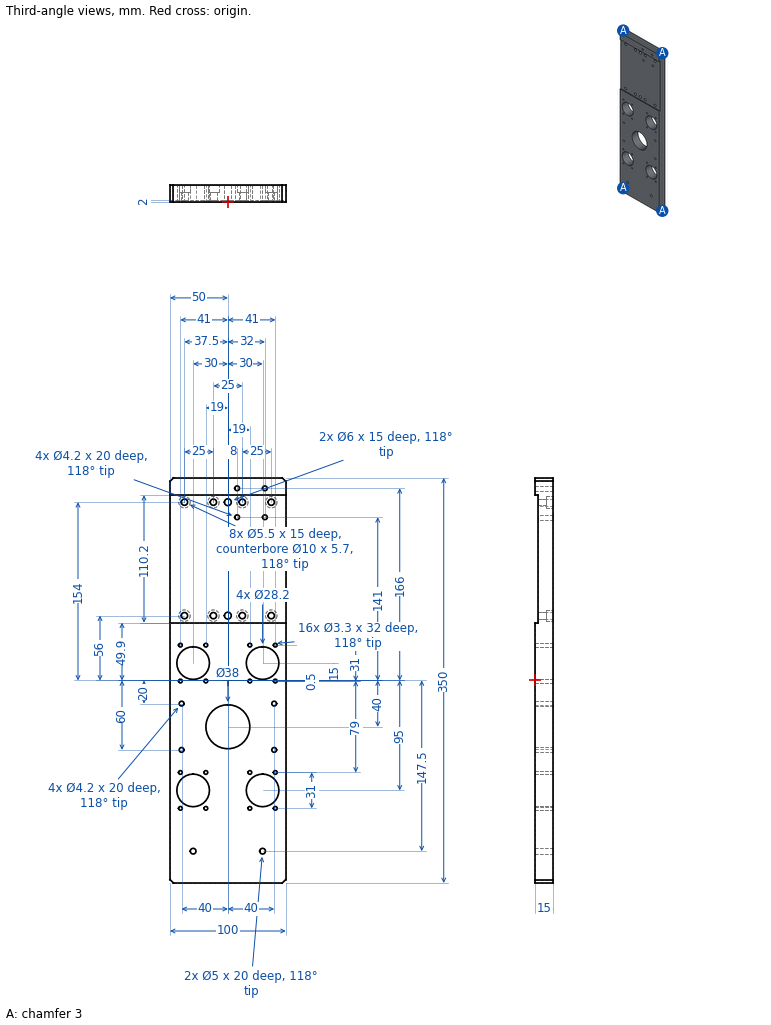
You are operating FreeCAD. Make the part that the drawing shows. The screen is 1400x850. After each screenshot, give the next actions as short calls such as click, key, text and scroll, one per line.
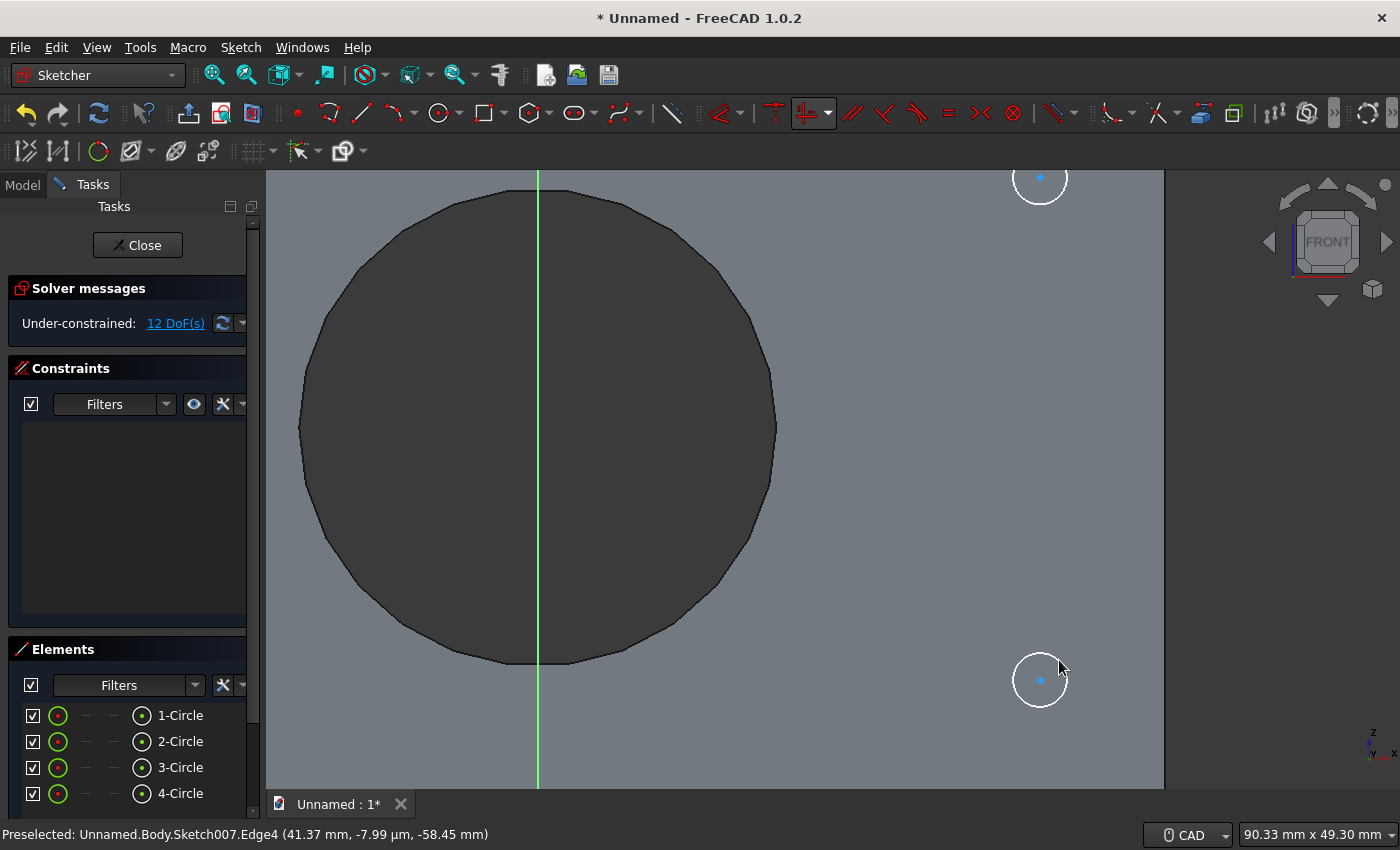
scroll(1040, 679, down, 3)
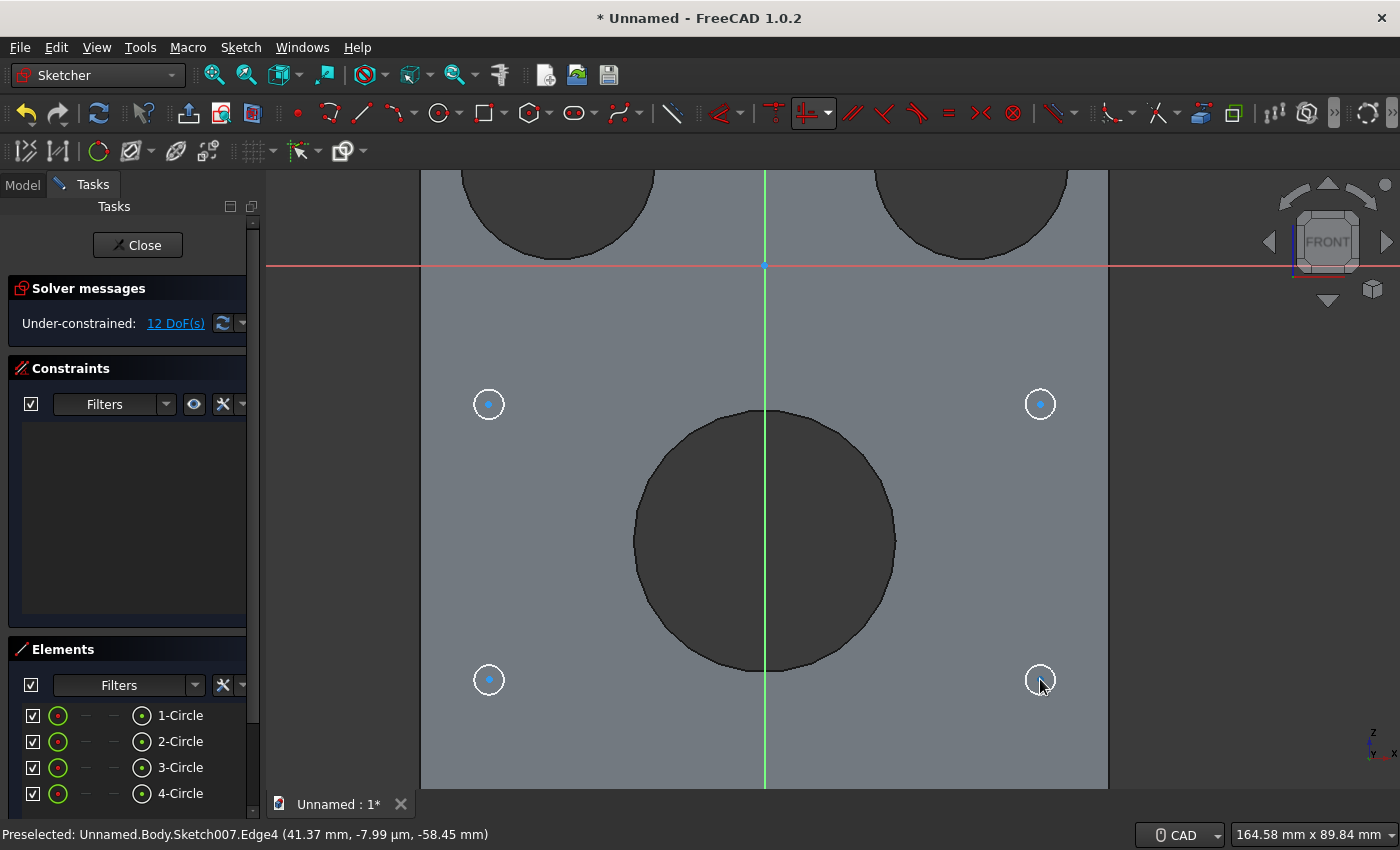
click(499, 394)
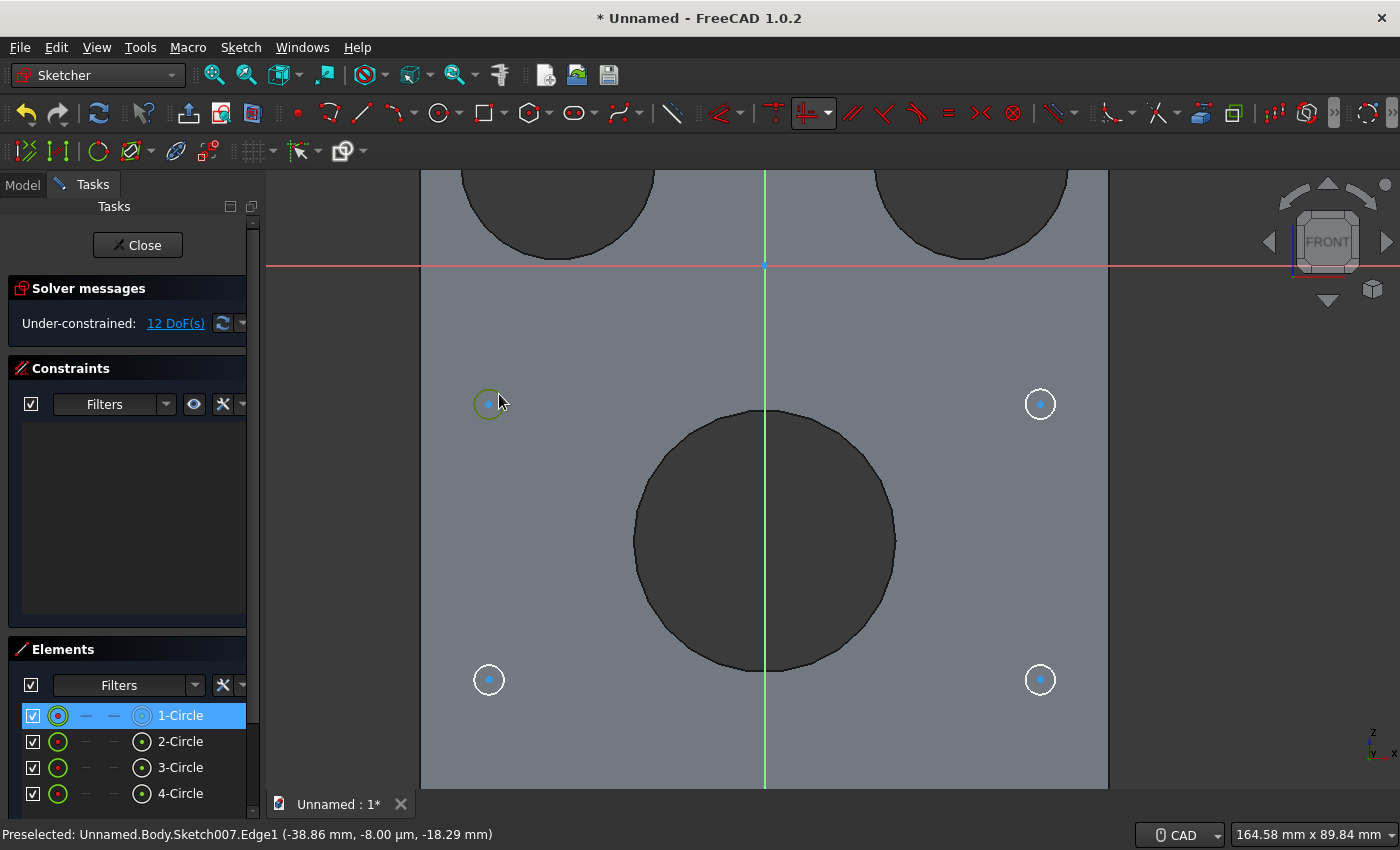
click(1051, 394)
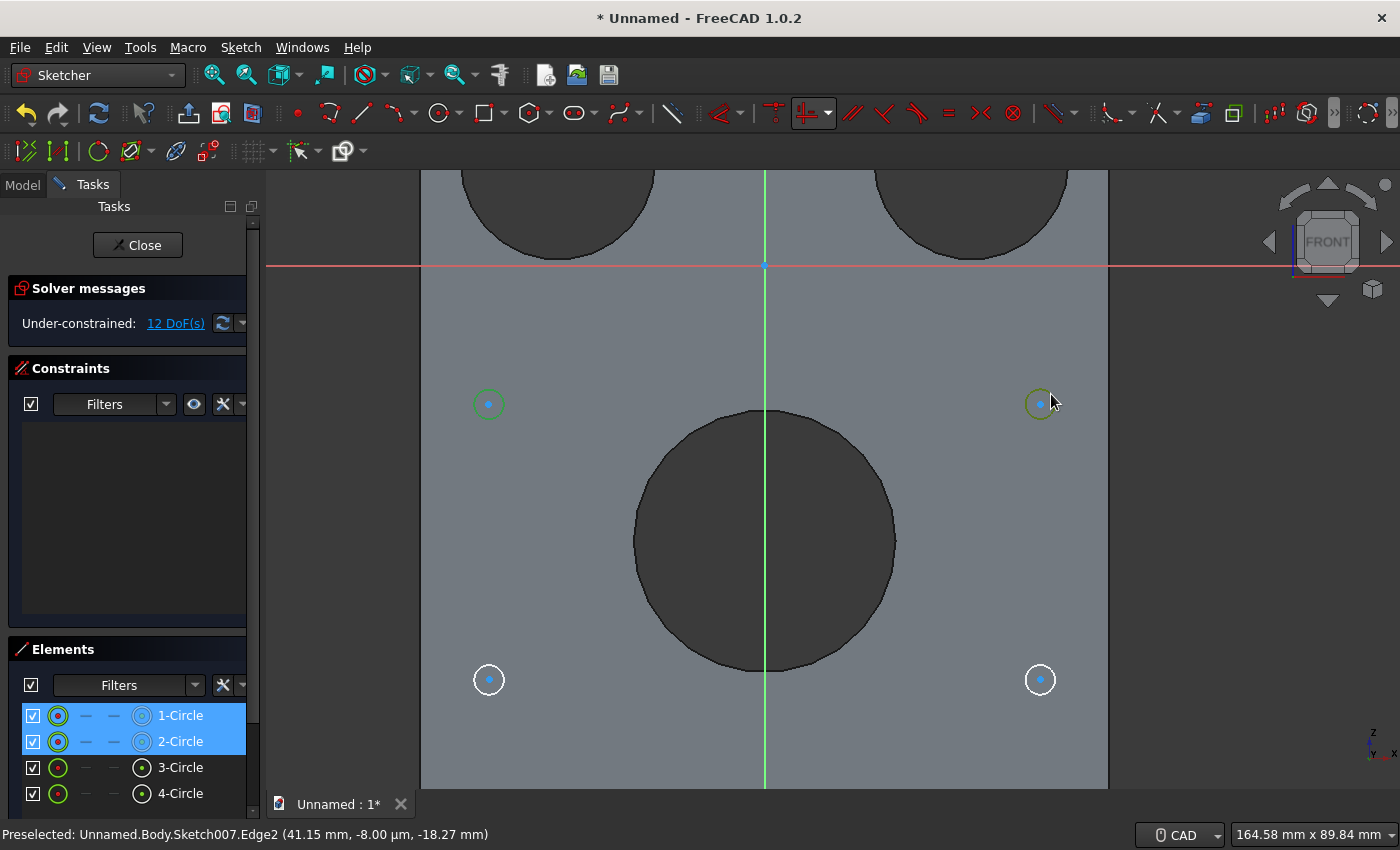
click(499, 669)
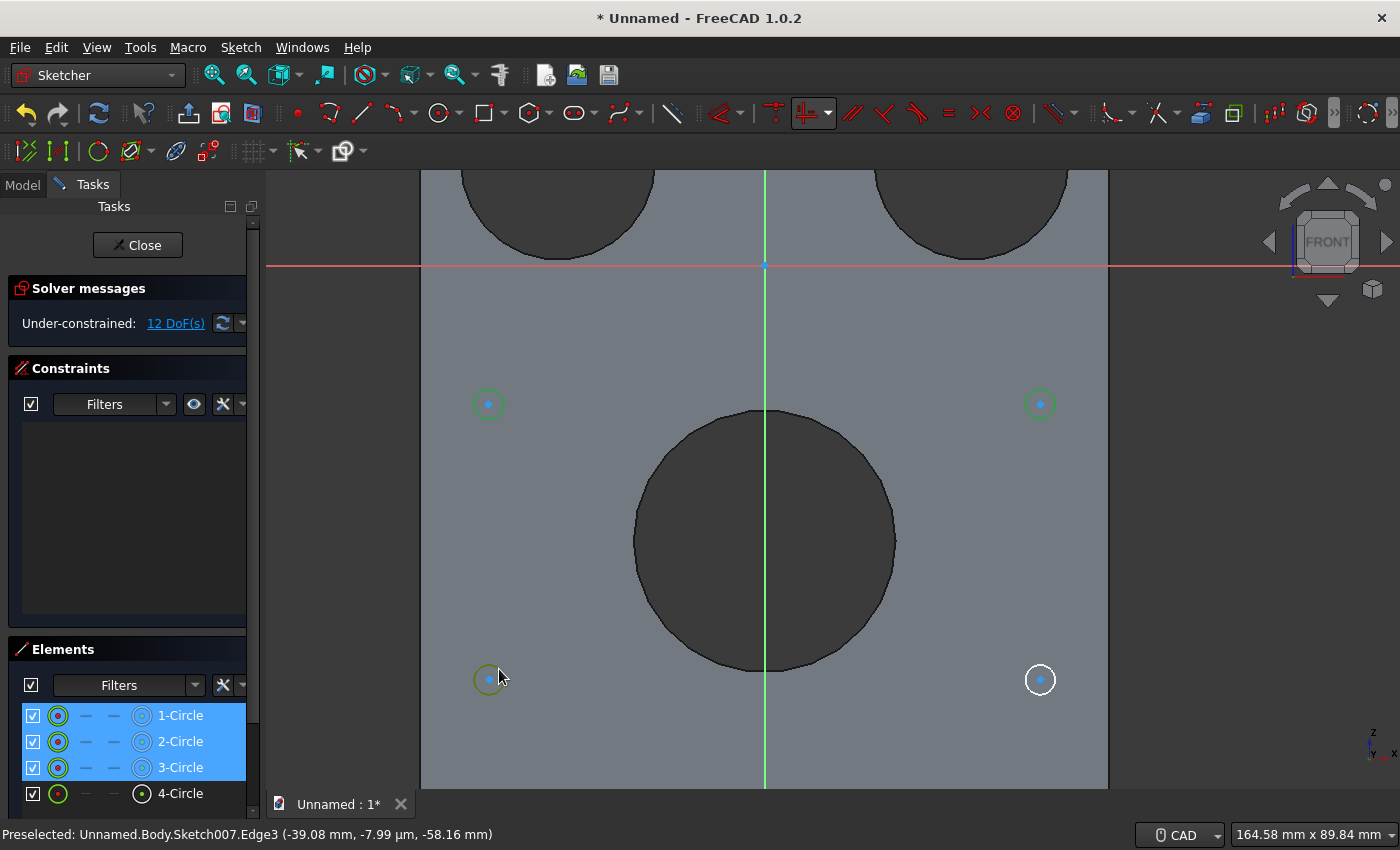
click(1051, 669)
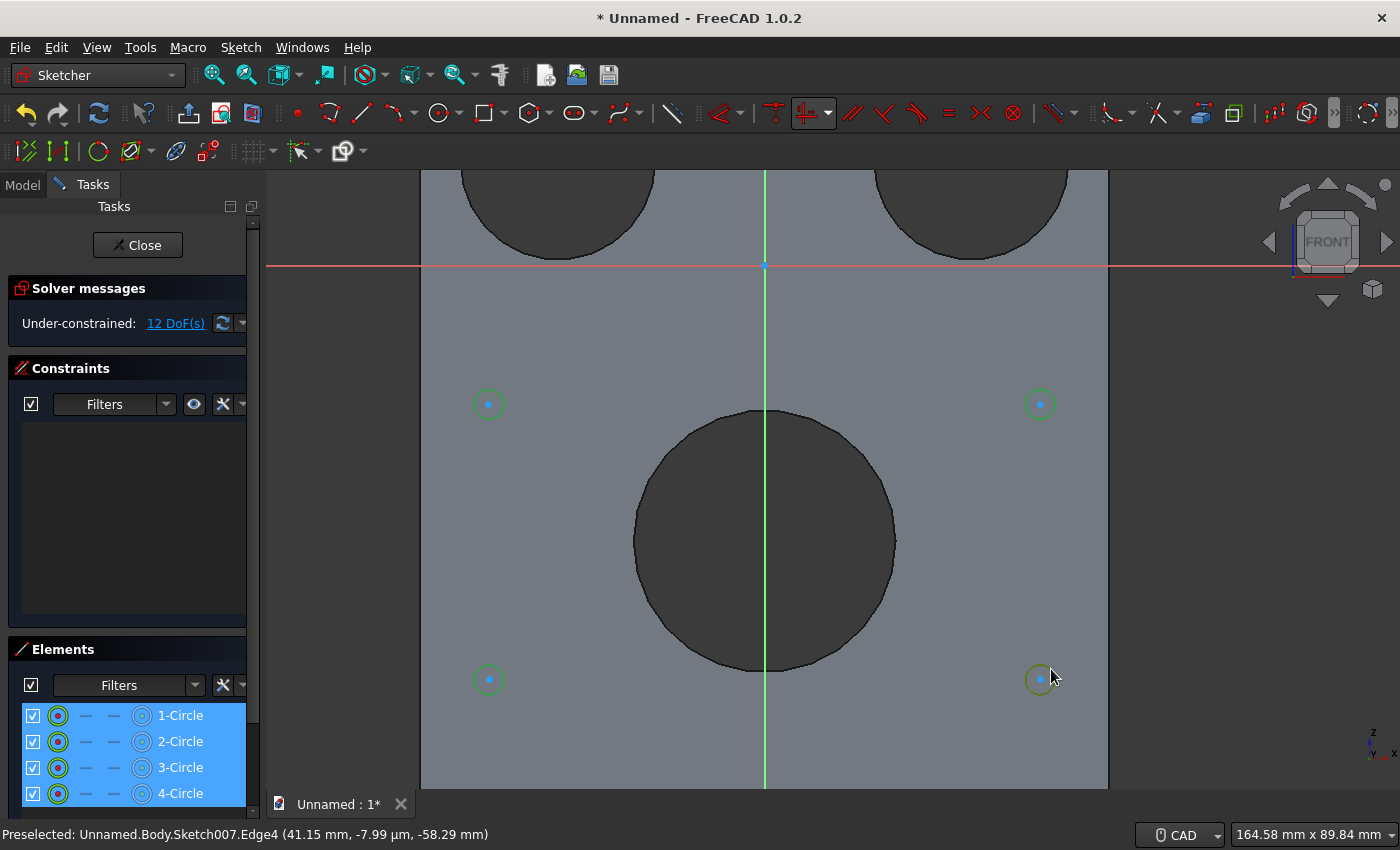
key(e)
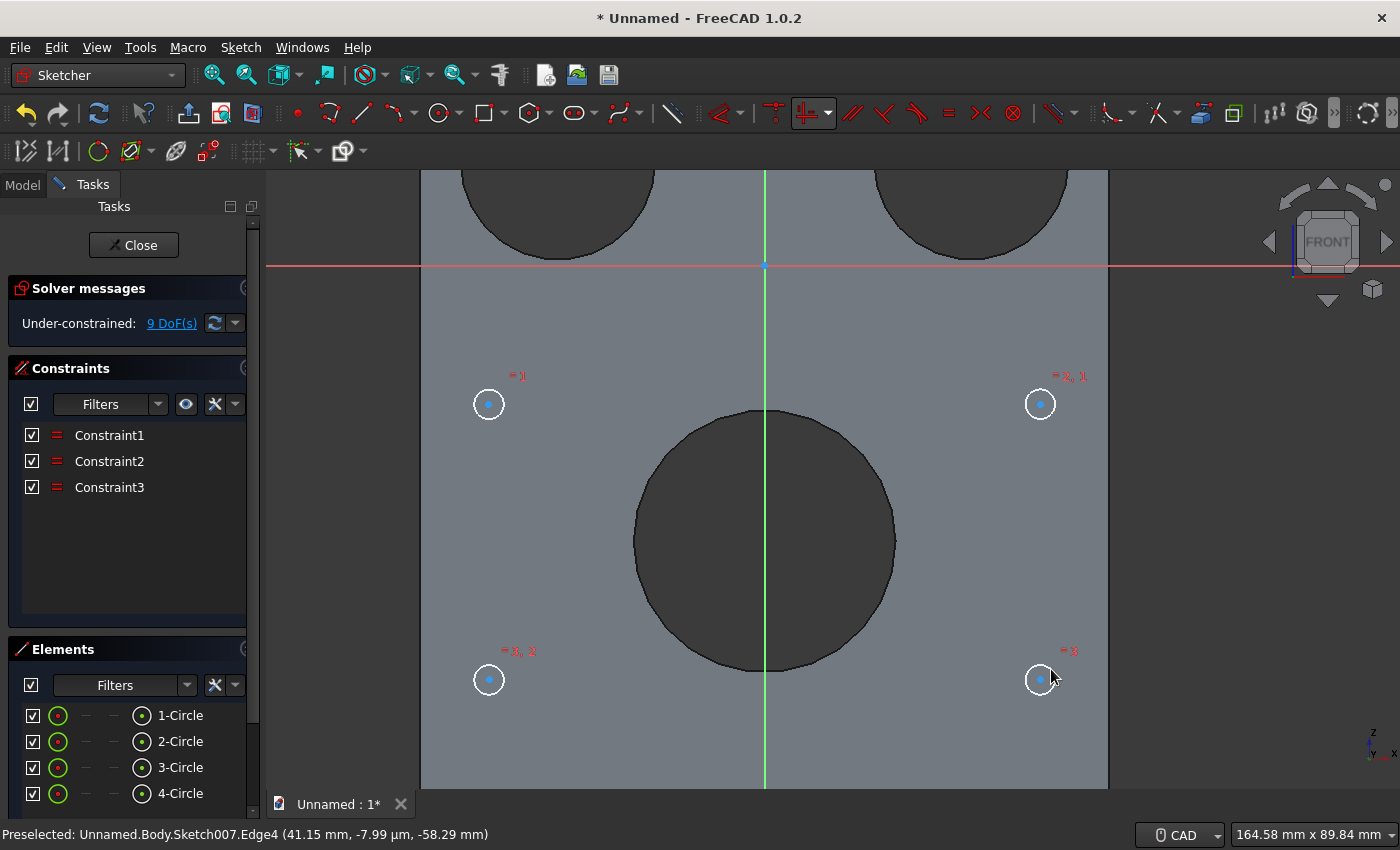
click(489, 404)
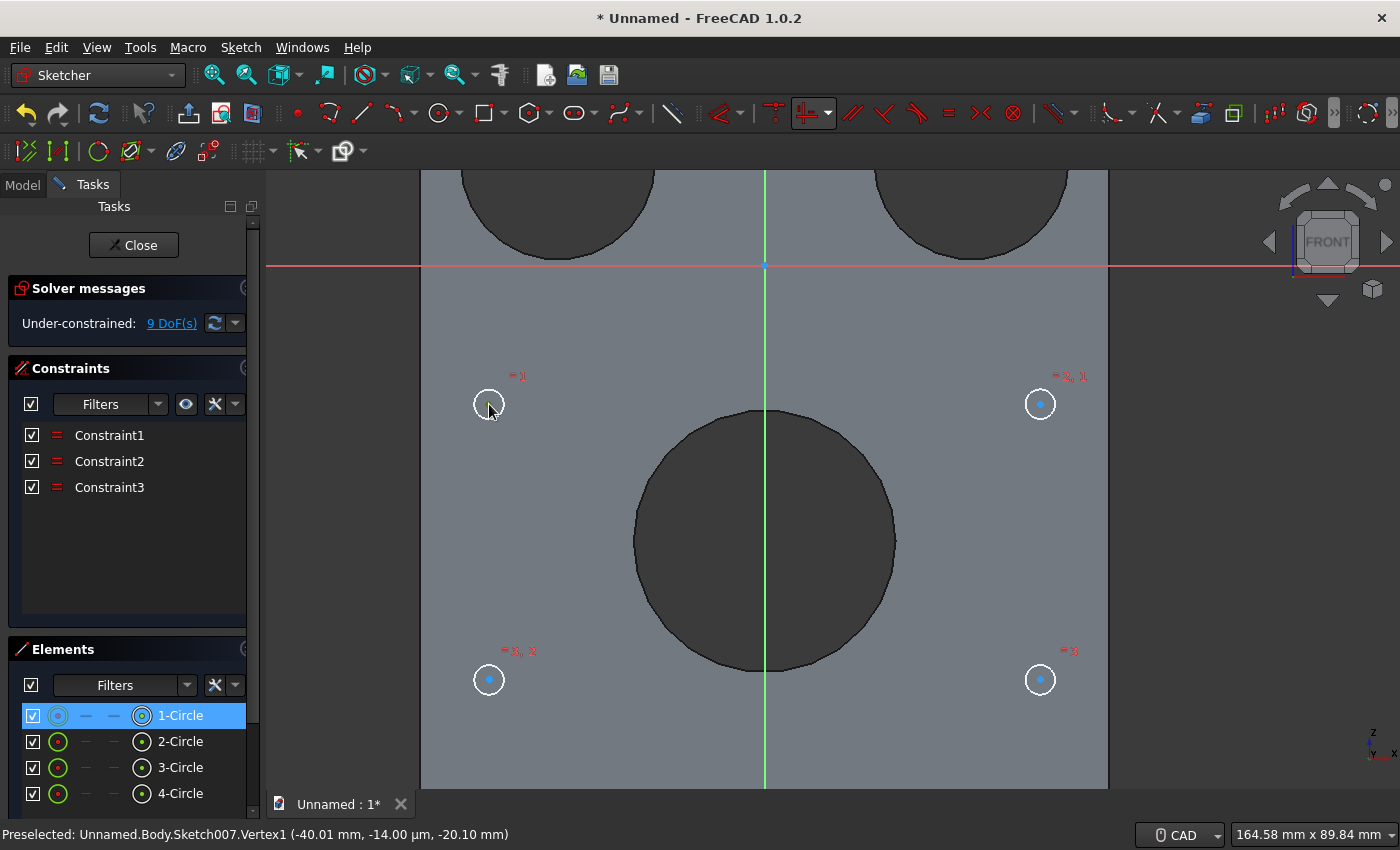
click(1040, 404)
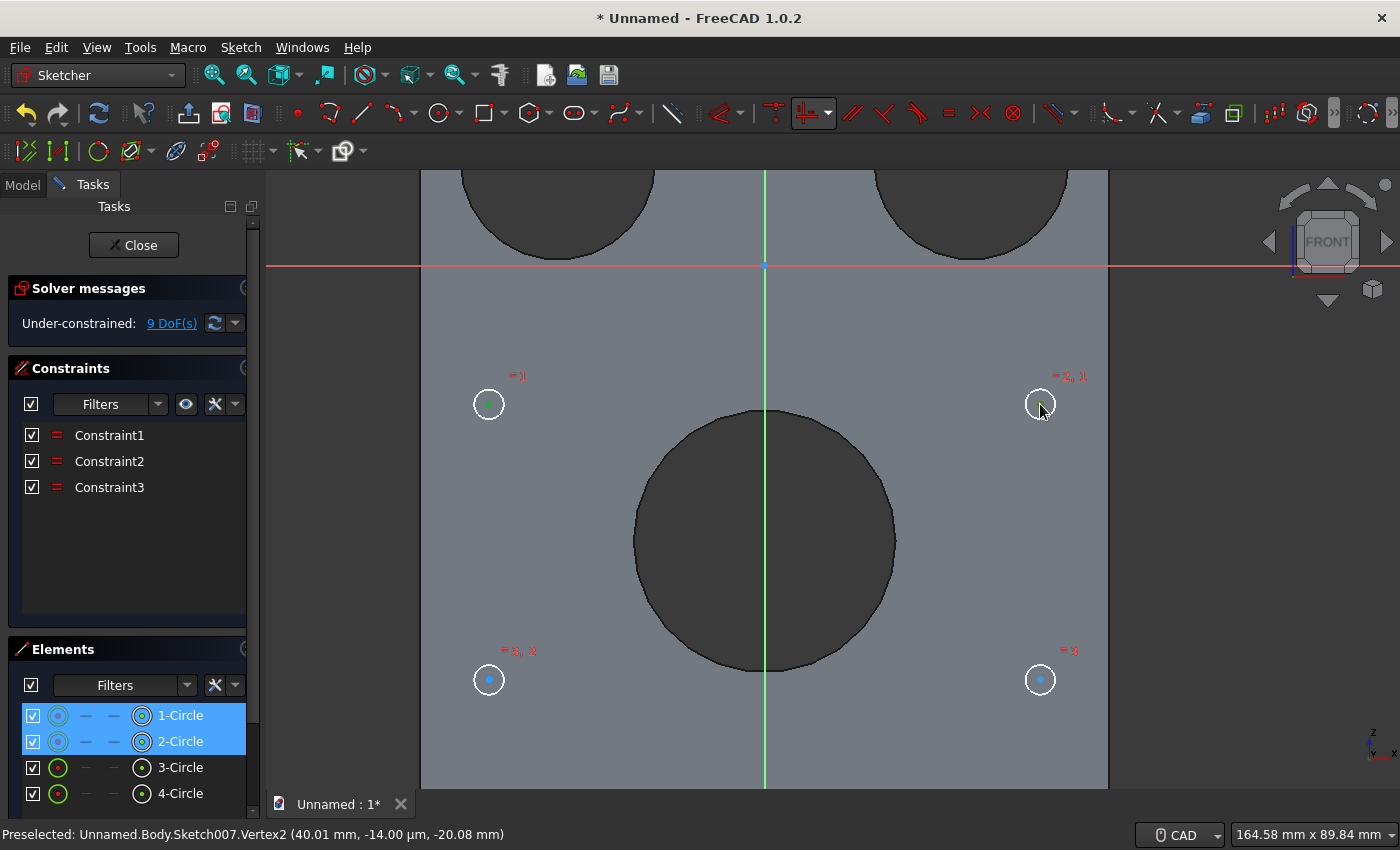
key(h)